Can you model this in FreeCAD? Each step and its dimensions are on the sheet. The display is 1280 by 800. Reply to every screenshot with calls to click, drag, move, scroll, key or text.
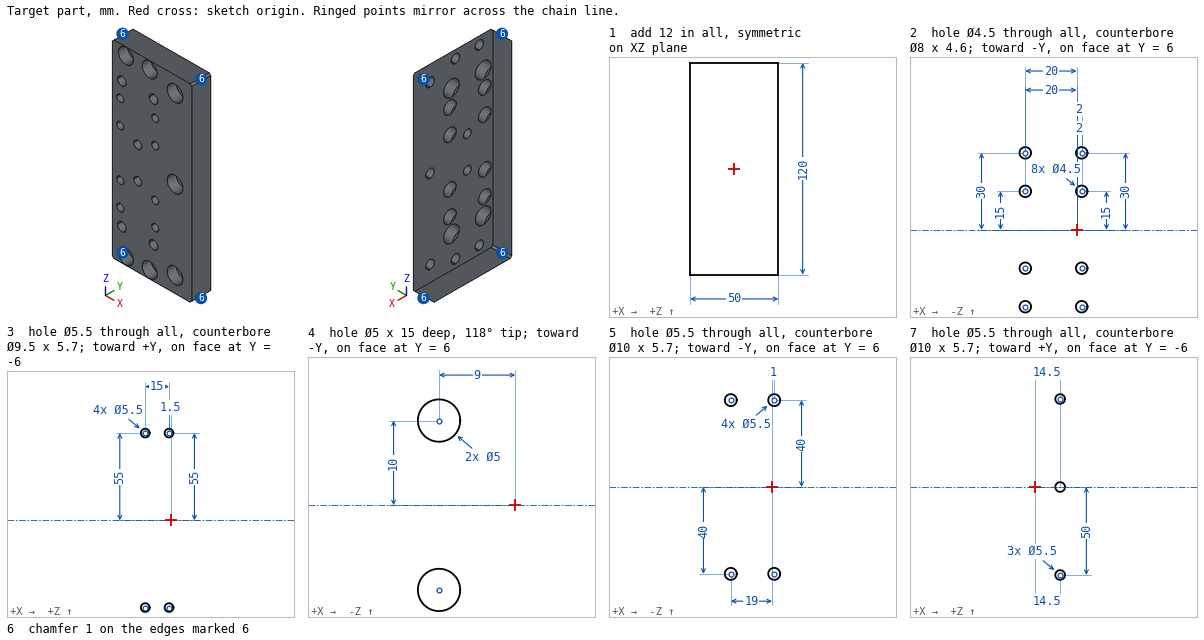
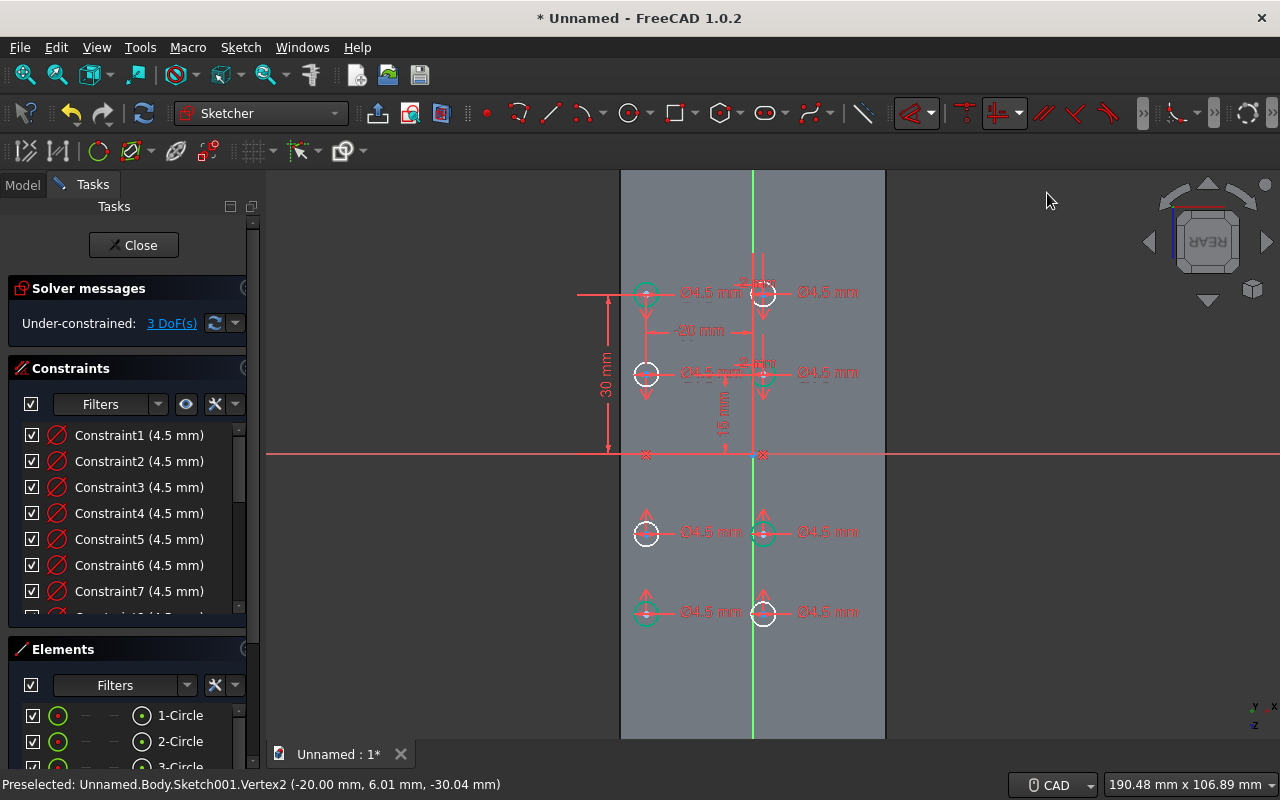
click(763, 294)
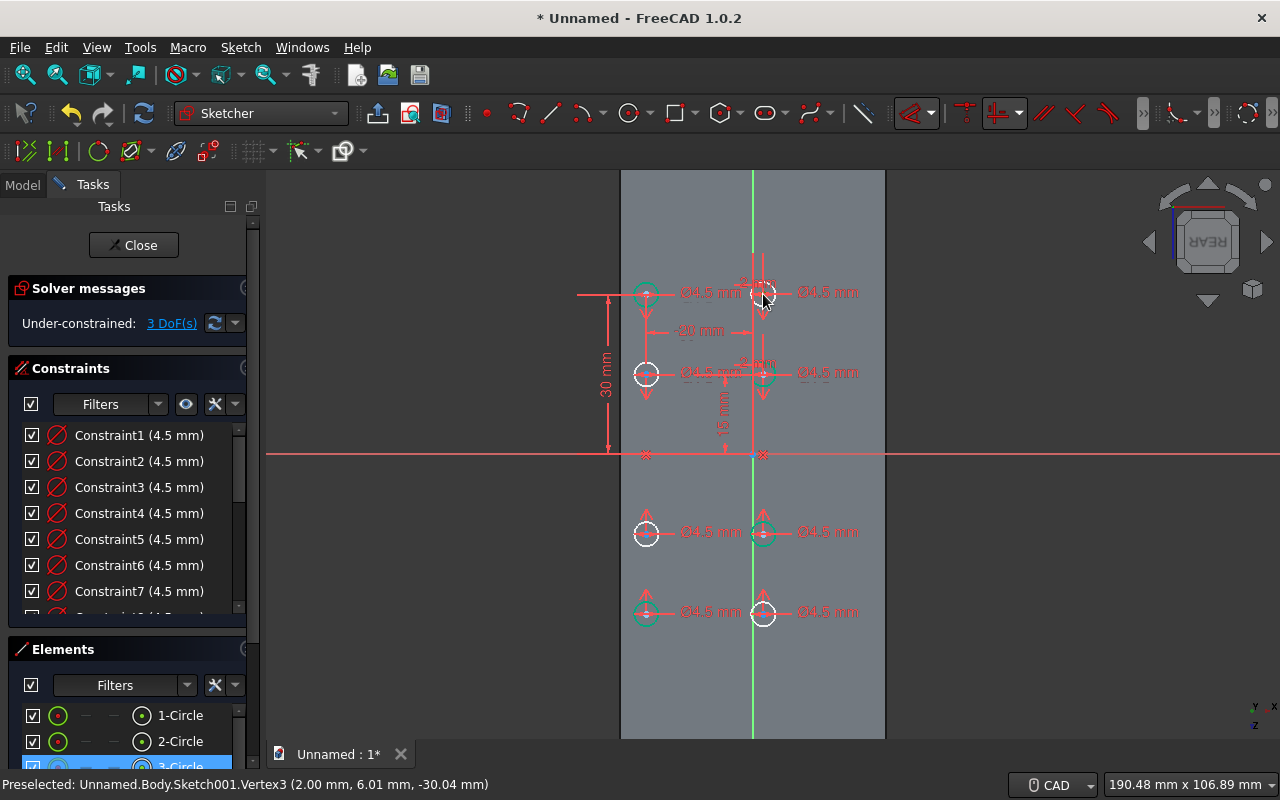
click(934, 114)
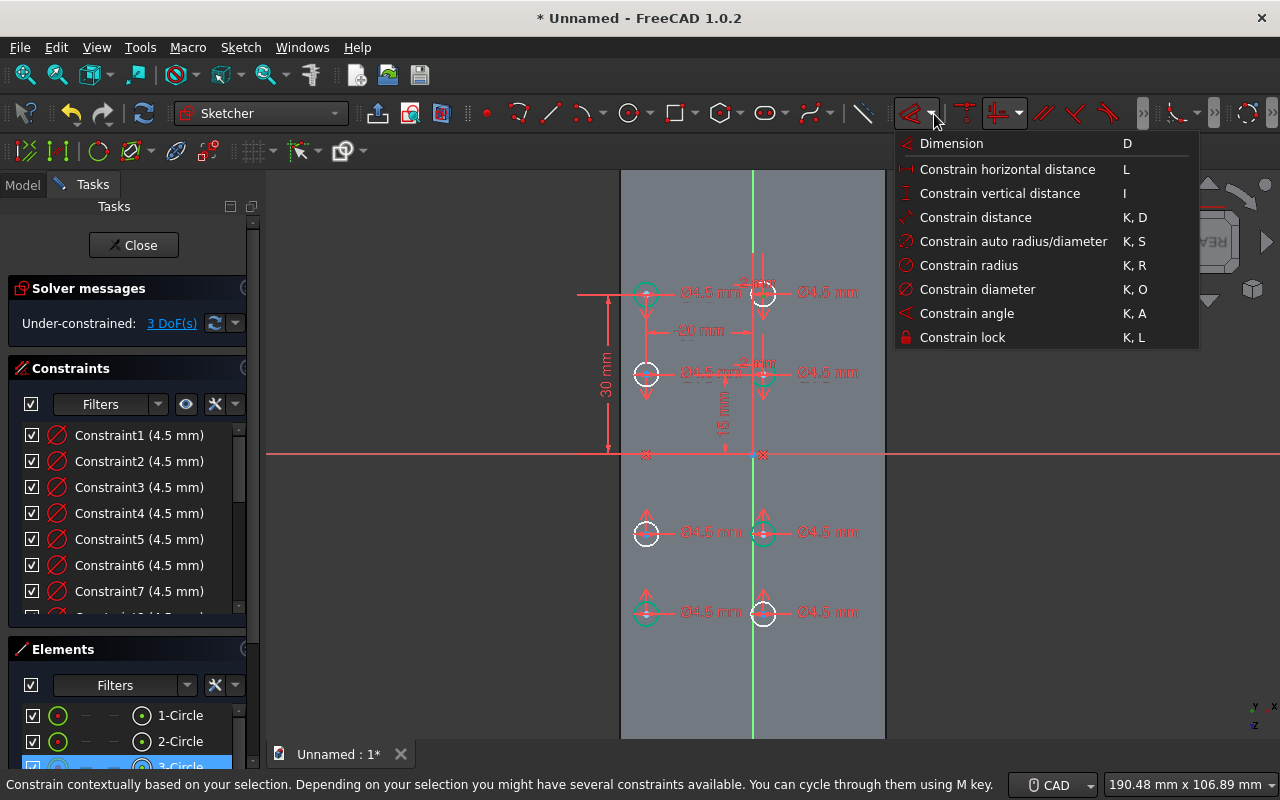
click(1047, 193)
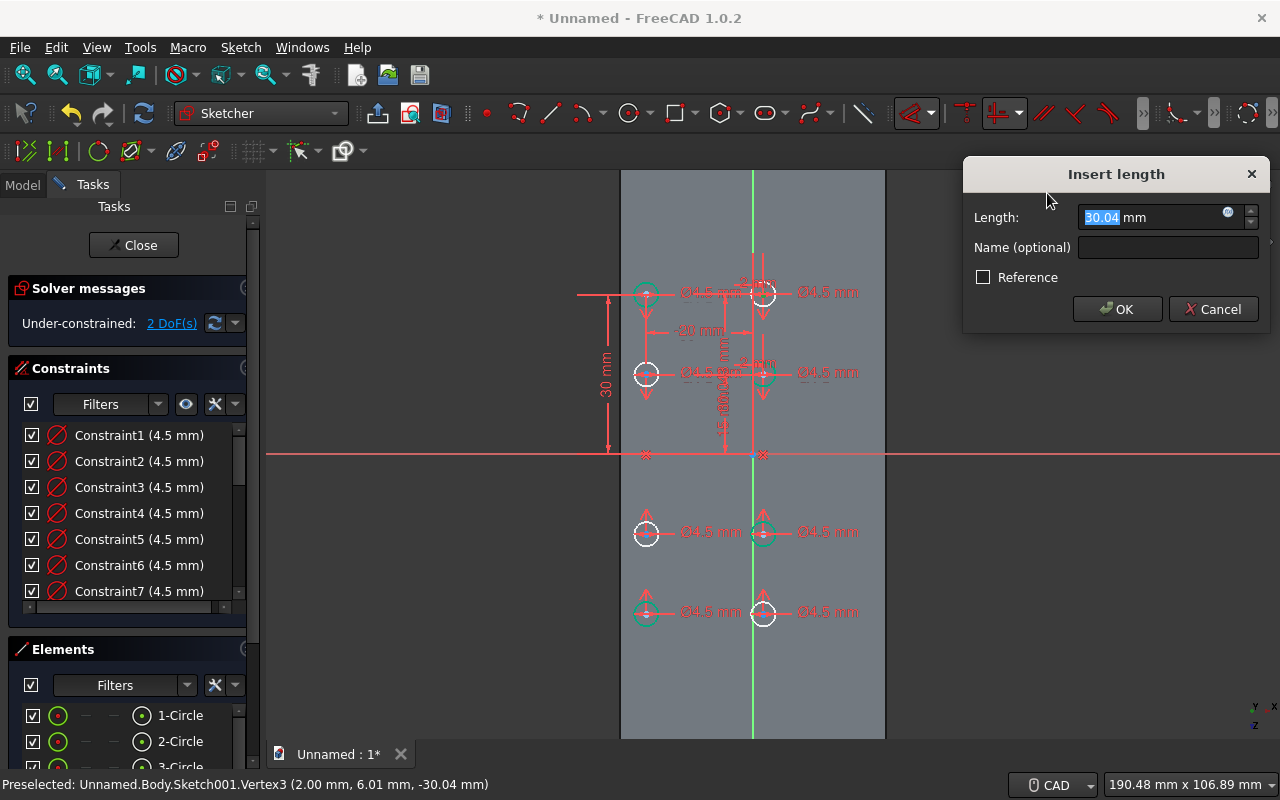
text(30)
key(Return)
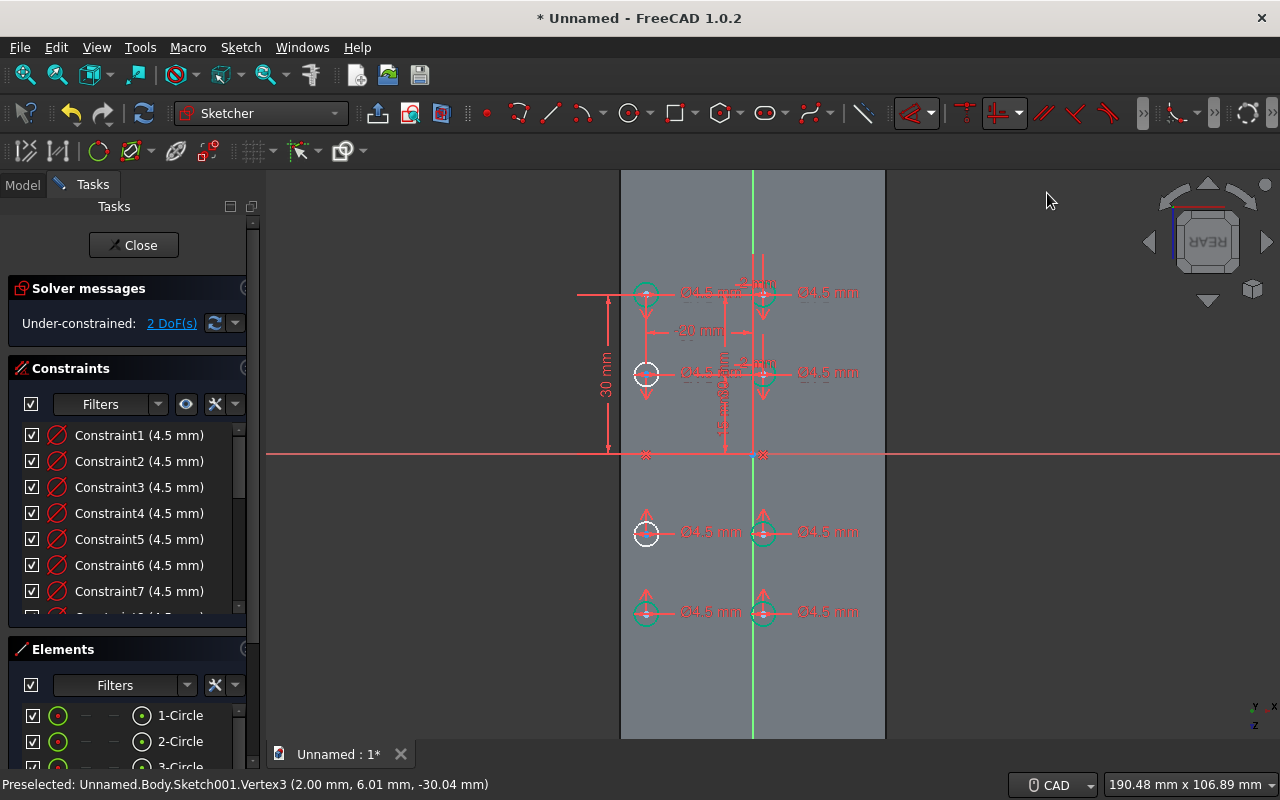
click(646, 375)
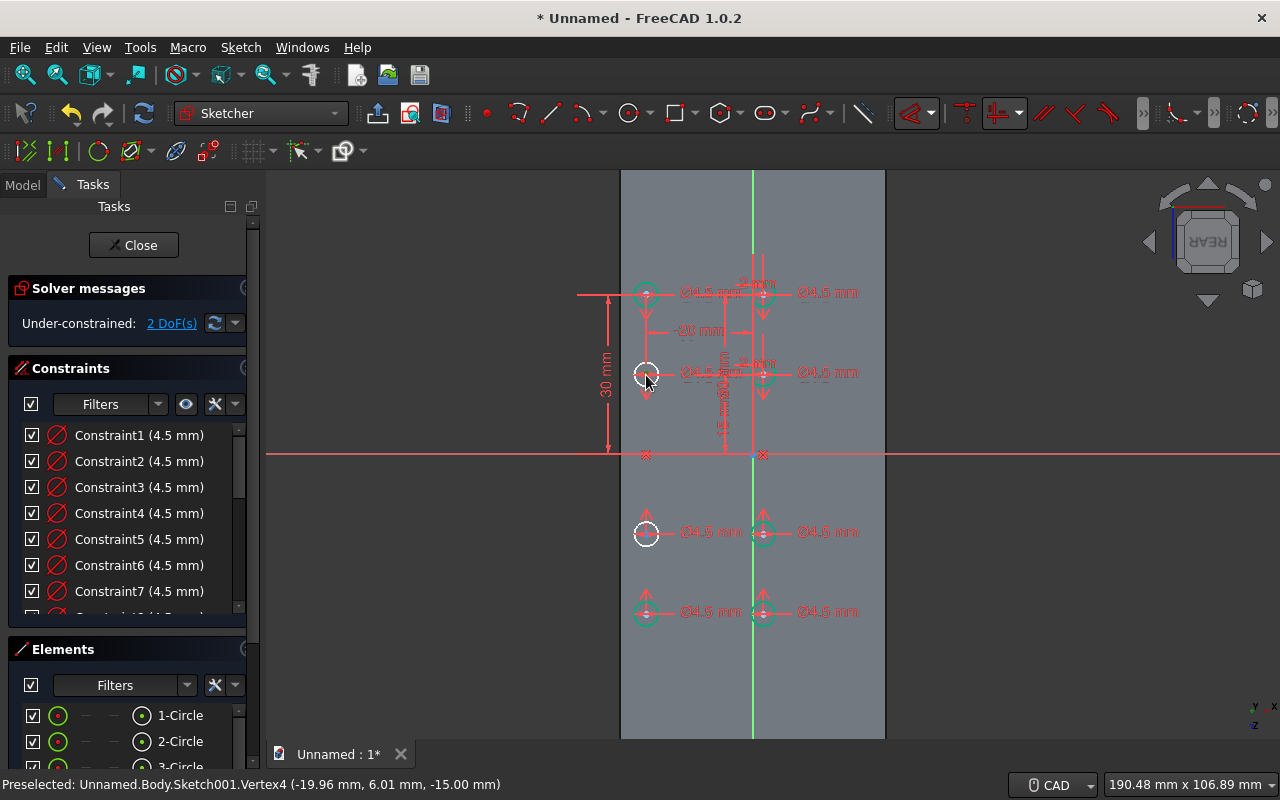
key(l)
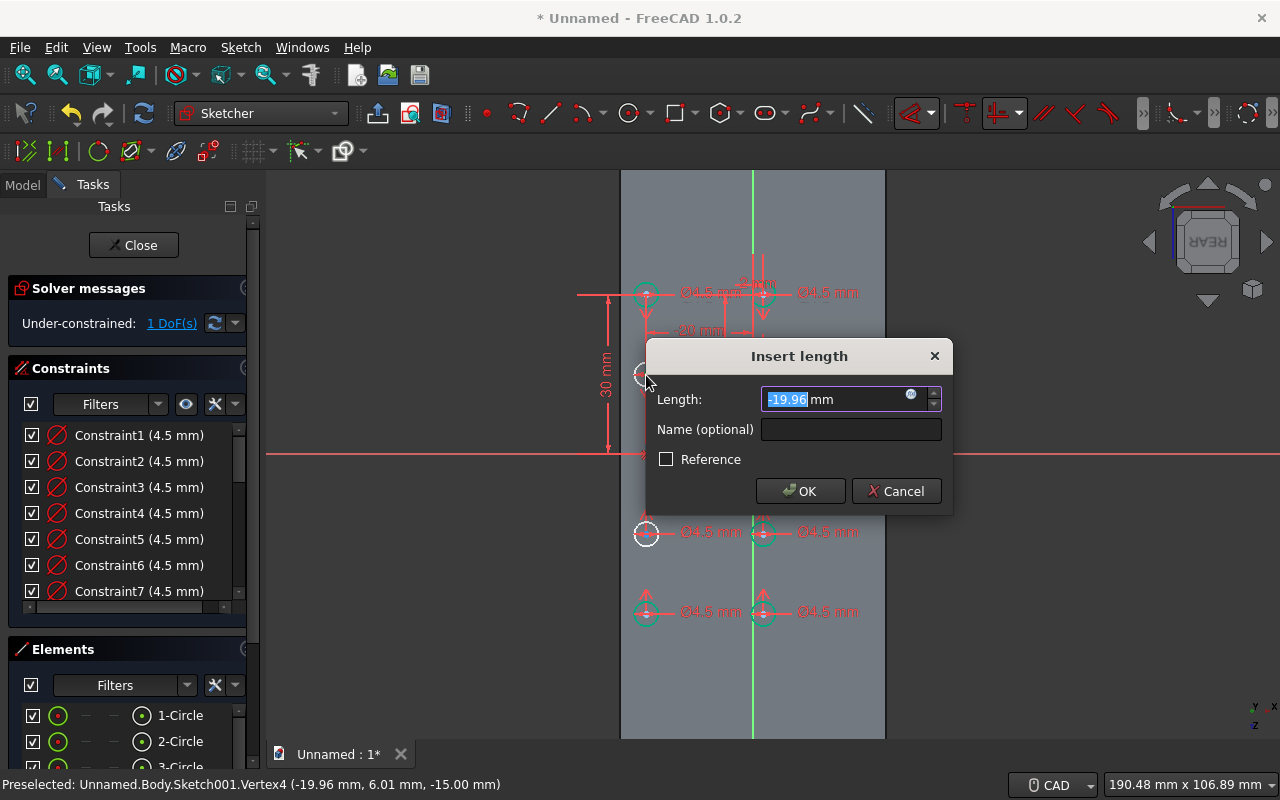
text(-20)
key(Return)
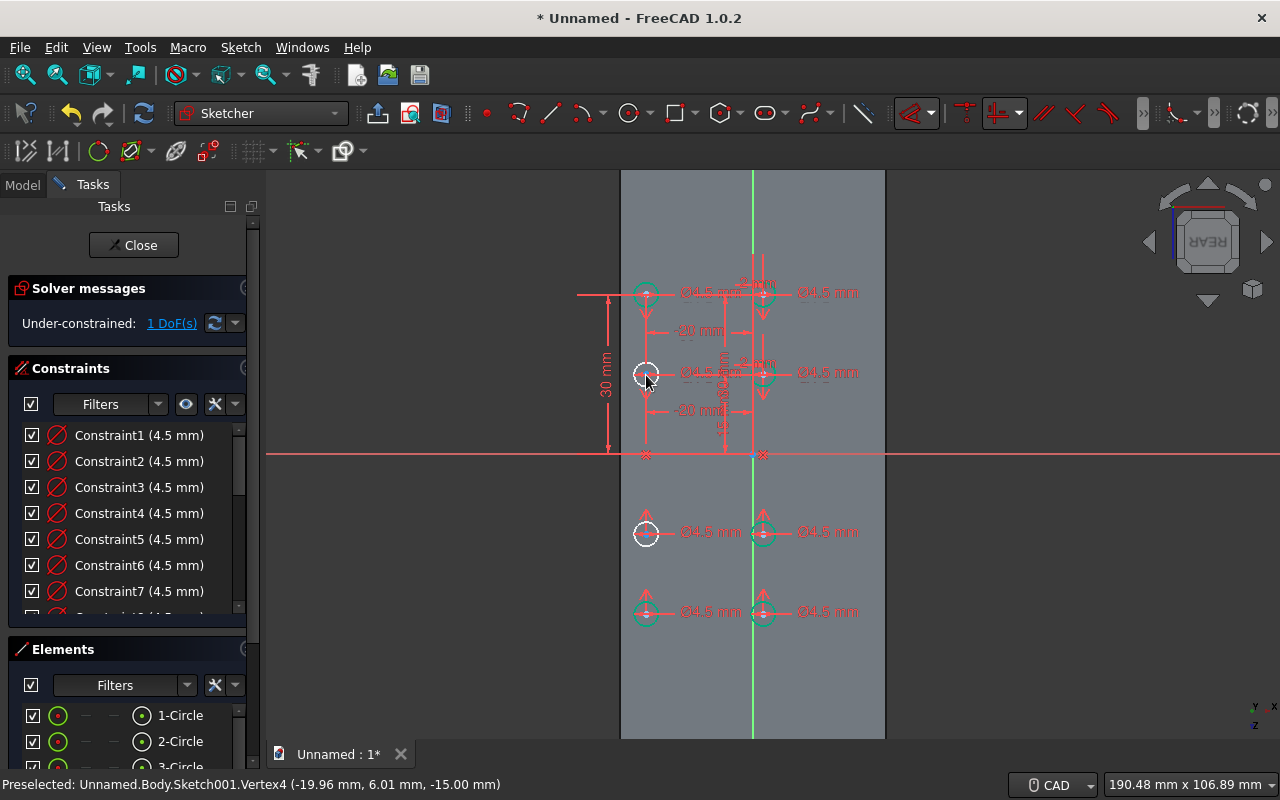
click(646, 375)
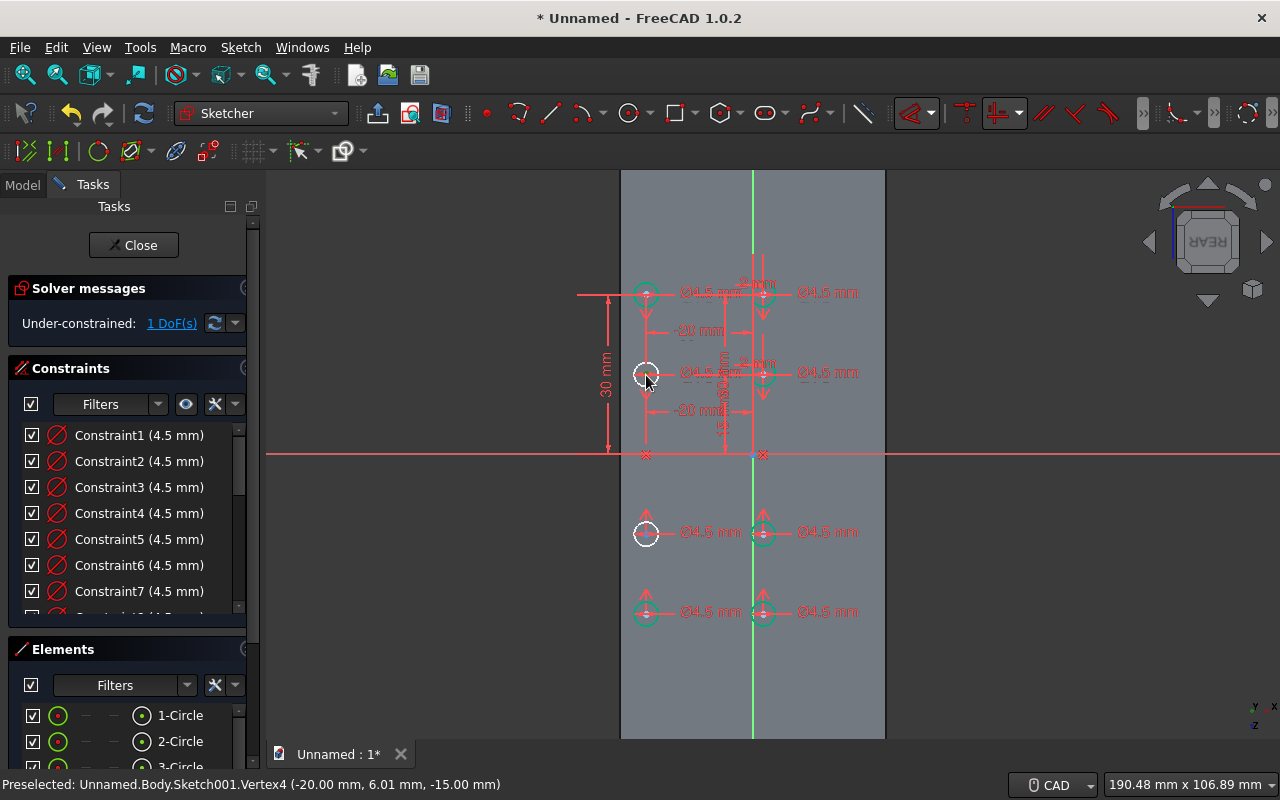
key(i)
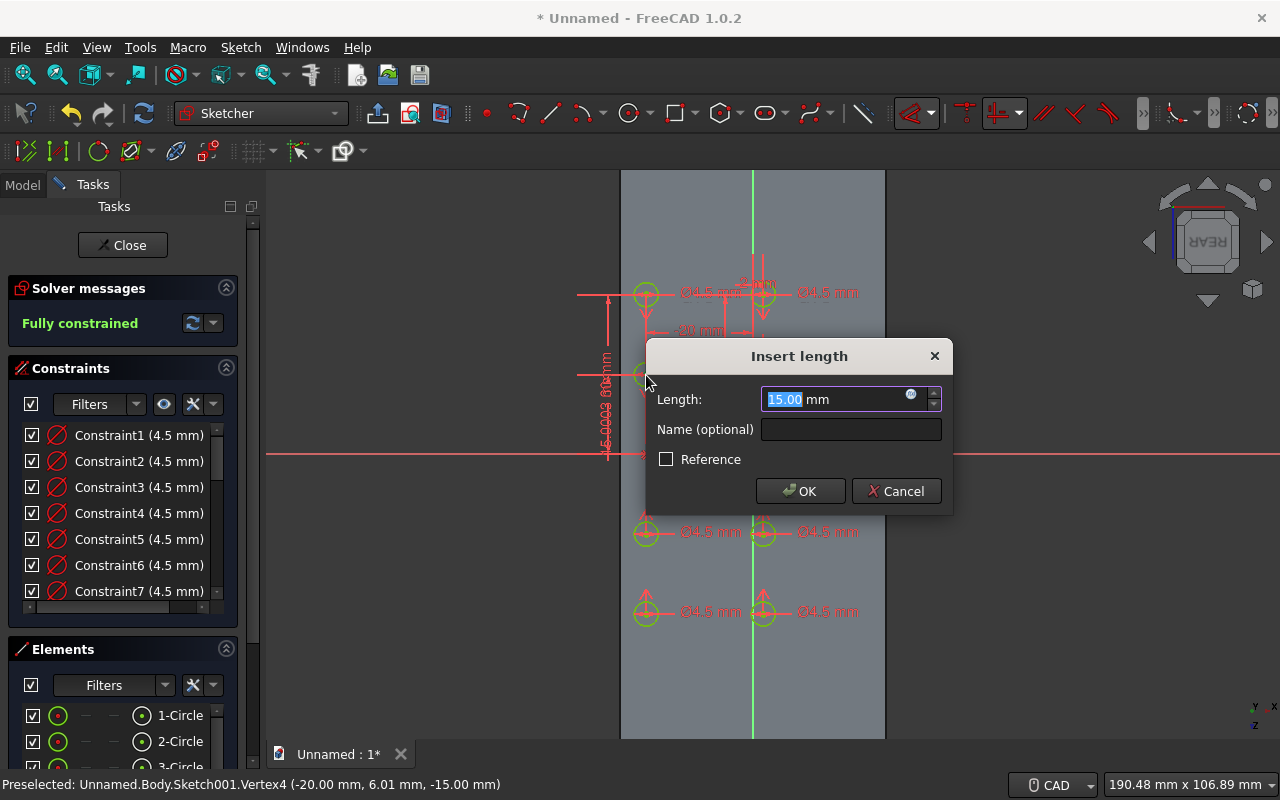
text(15)
key(Return)